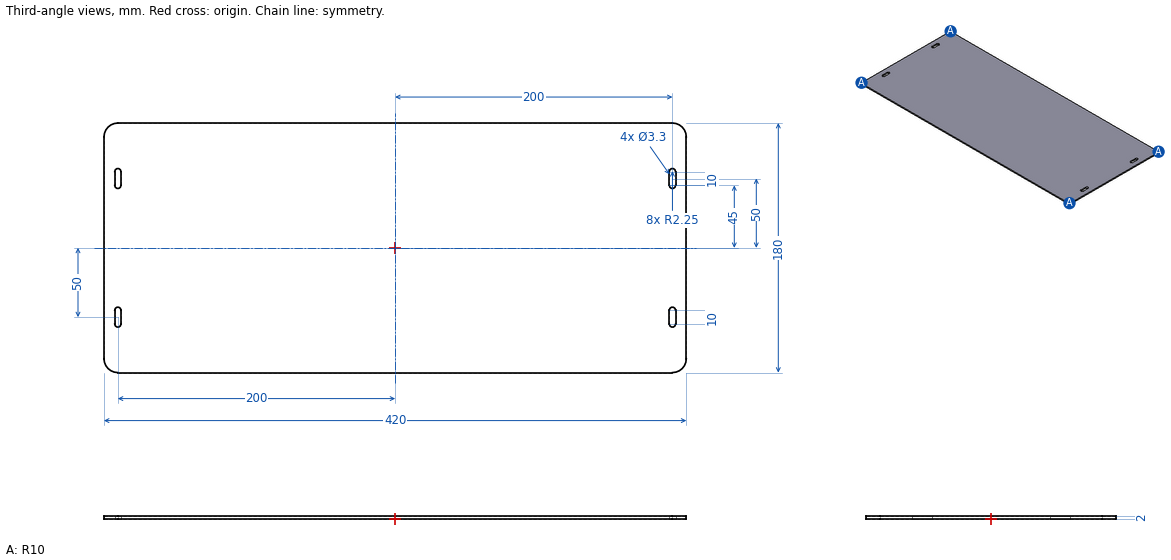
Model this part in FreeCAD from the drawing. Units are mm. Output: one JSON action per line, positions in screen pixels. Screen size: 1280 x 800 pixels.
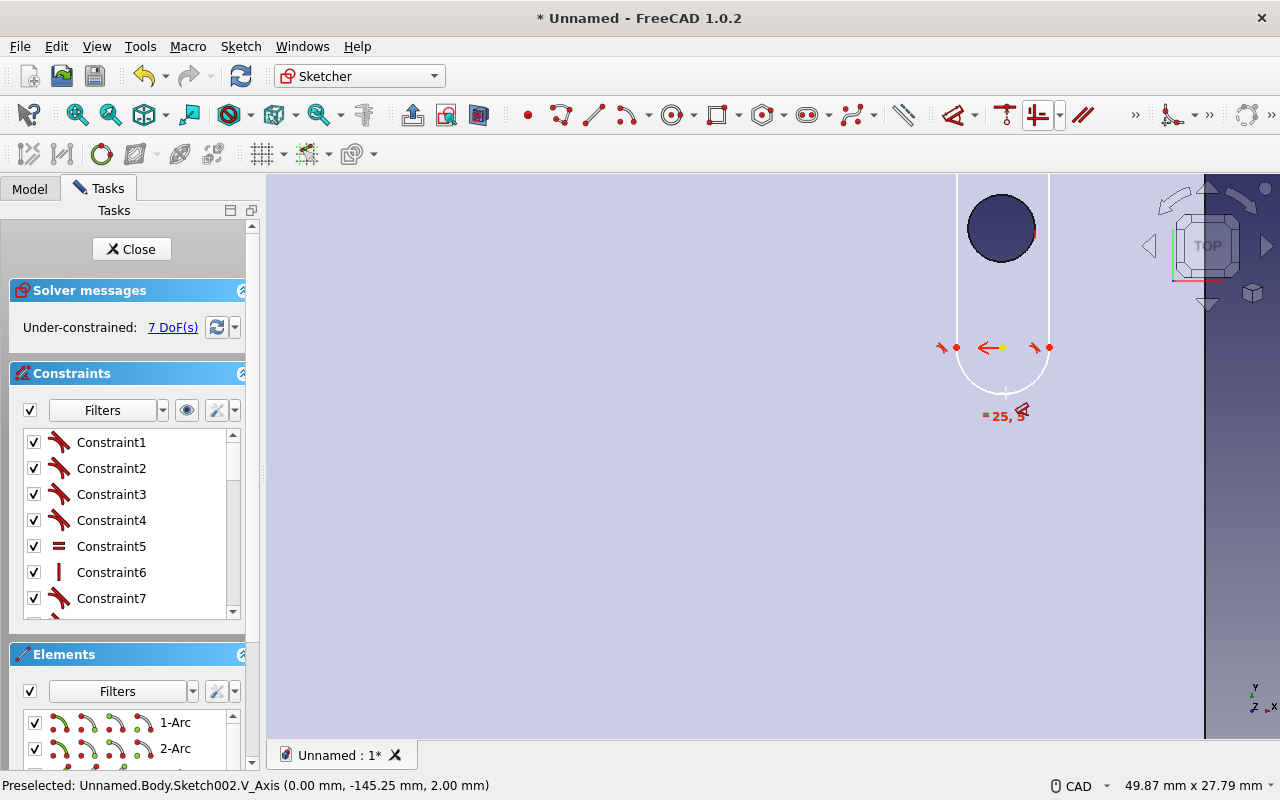
{"action": "left_click", "coordinate": [1003, 394]}
{"action": "left_click", "coordinate": [1003, 426]}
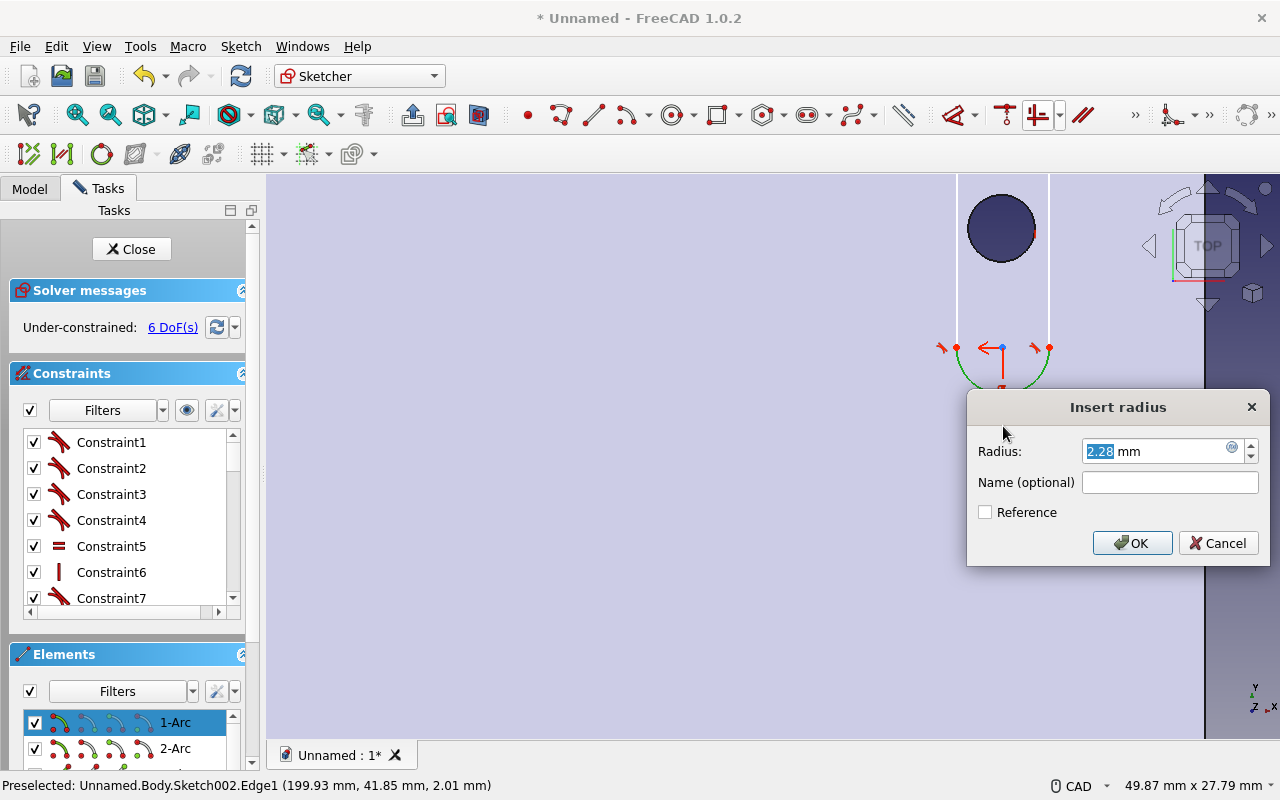
{"action": "type", "text": "2.25"}
{"action": "key", "text": "Return"}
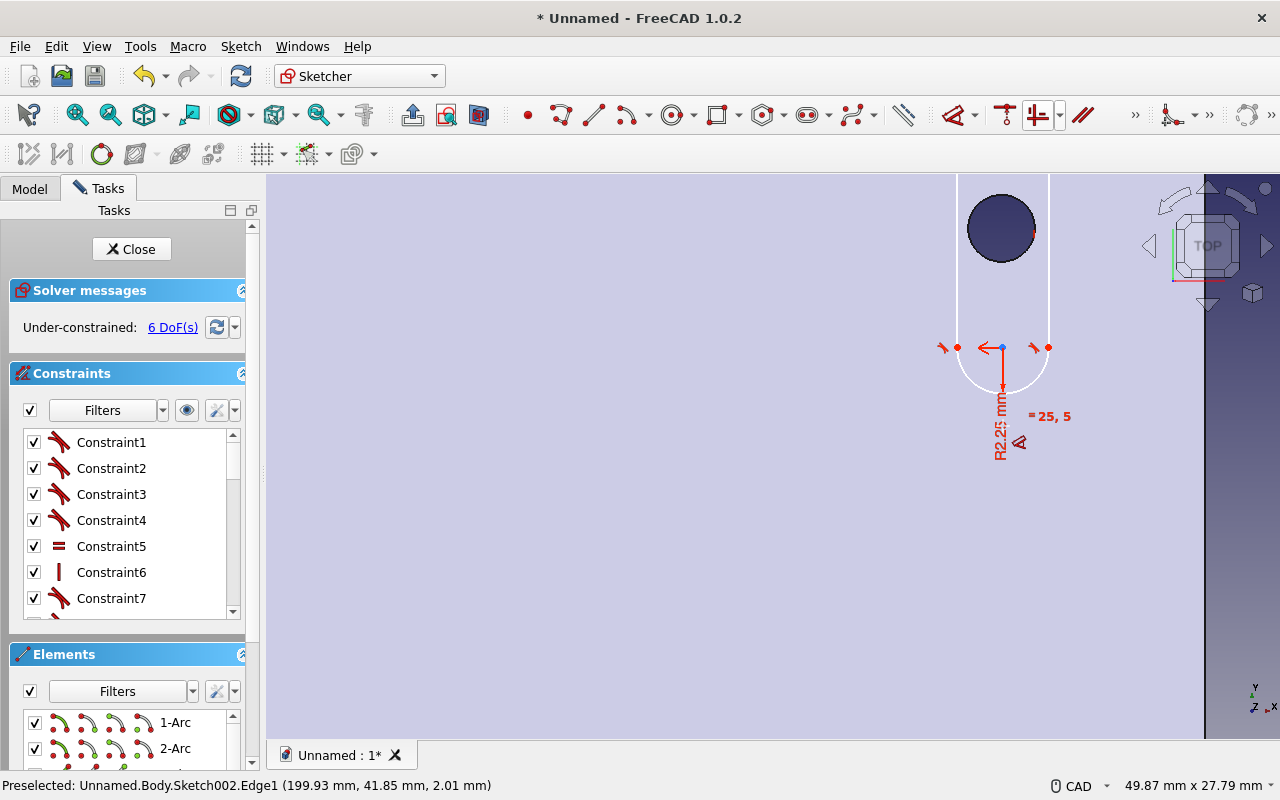
{"action": "scroll", "coordinate": [1007, 393], "scroll_direction": "down", "scroll_amount": 13}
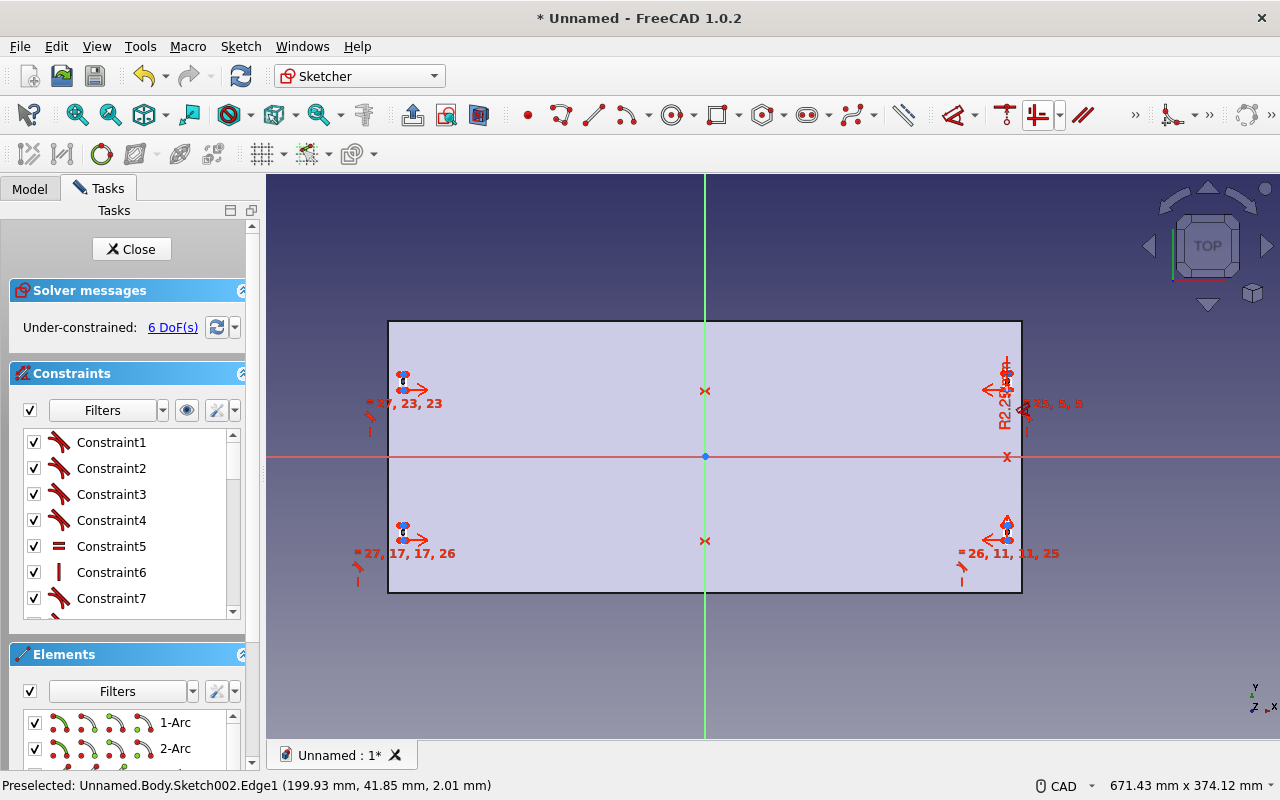
{"action": "scroll", "coordinate": [1004, 385], "scroll_direction": "up", "scroll_amount": 5}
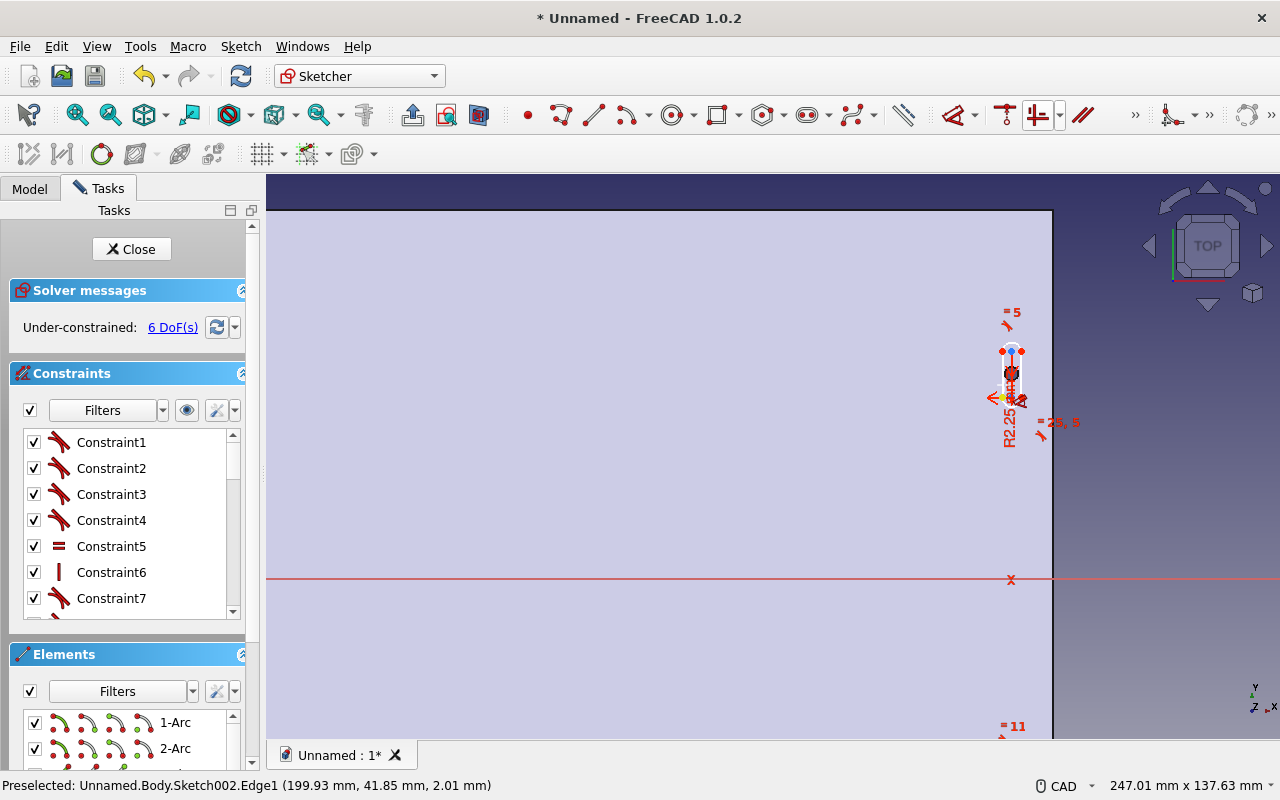
{"action": "left_click", "coordinate": [1003, 384]}
{"action": "left_click", "coordinate": [1037, 375]}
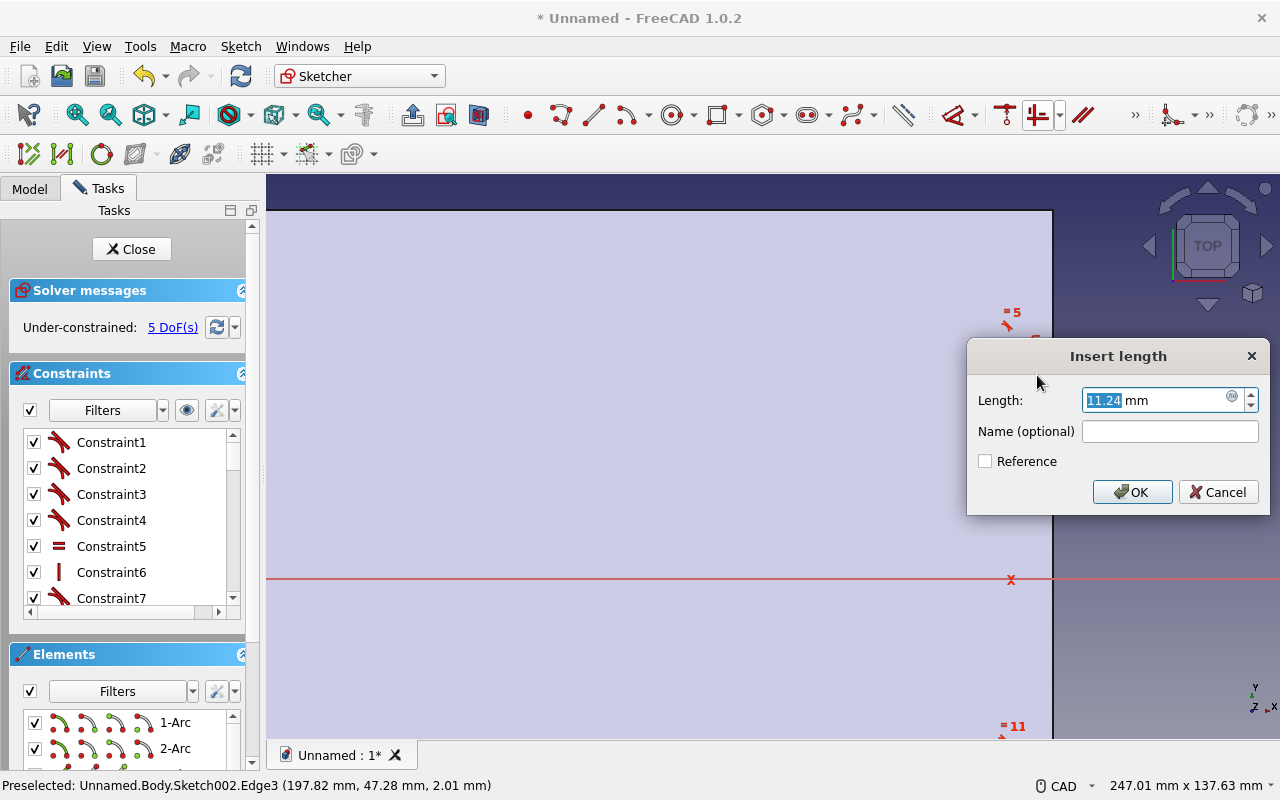
{"action": "type", "text": "10"}
{"action": "key", "text": "Return"}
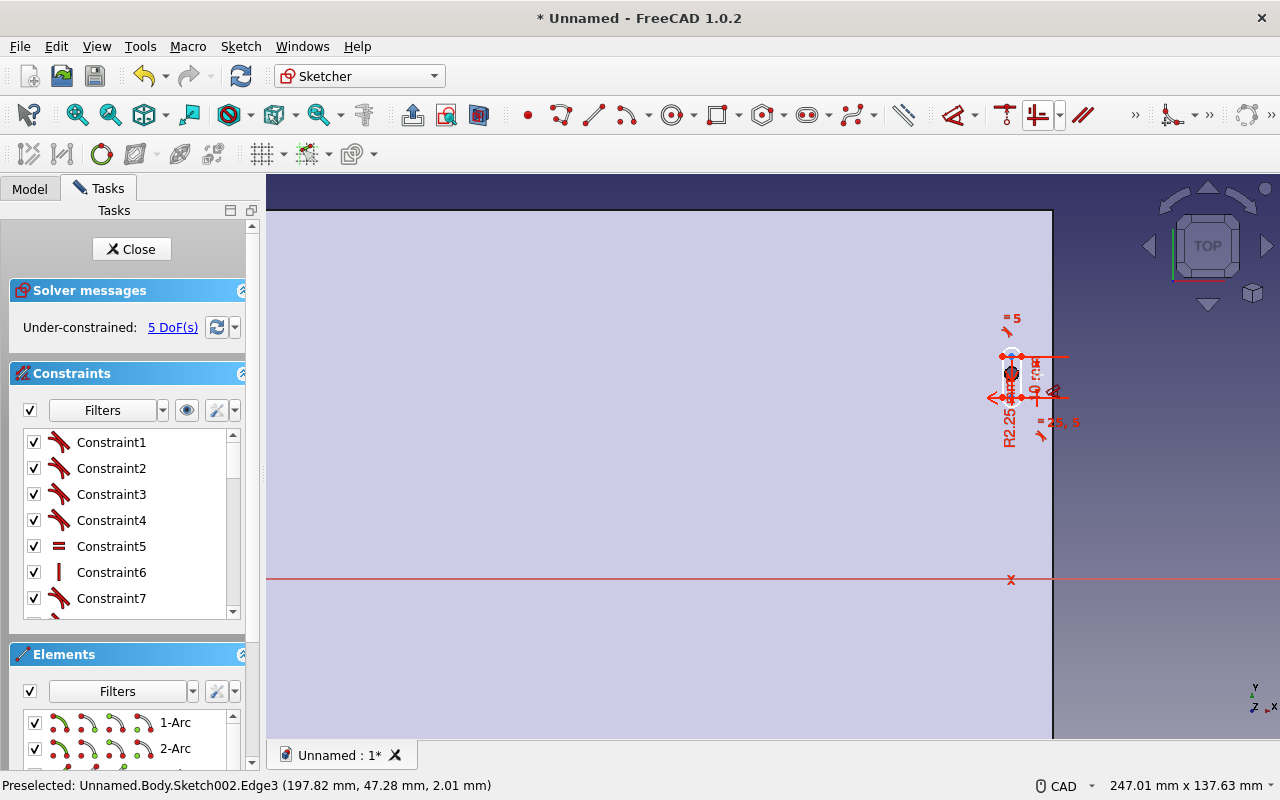
{"action": "scroll", "coordinate": [1004, 385], "scroll_direction": "down", "scroll_amount": 5}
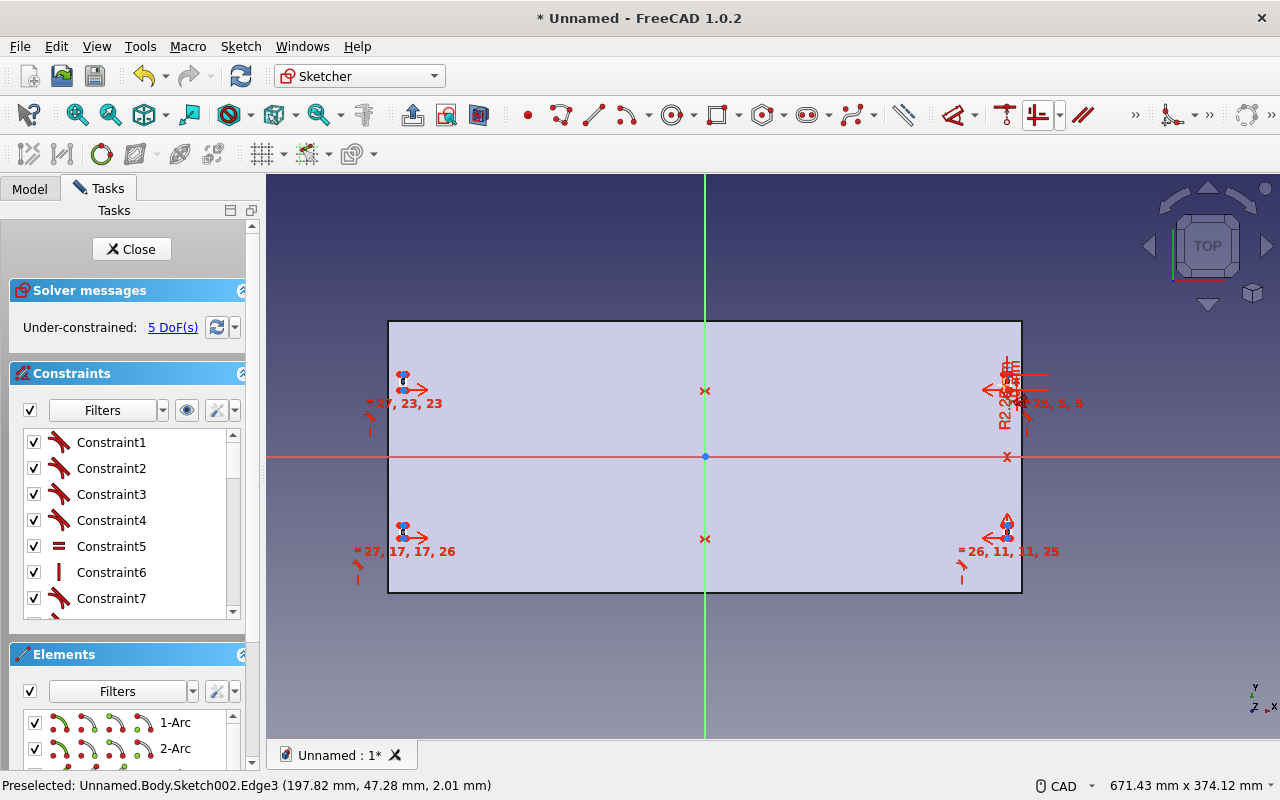
{"action": "scroll", "coordinate": [1004, 534], "scroll_direction": "up", "scroll_amount": 7}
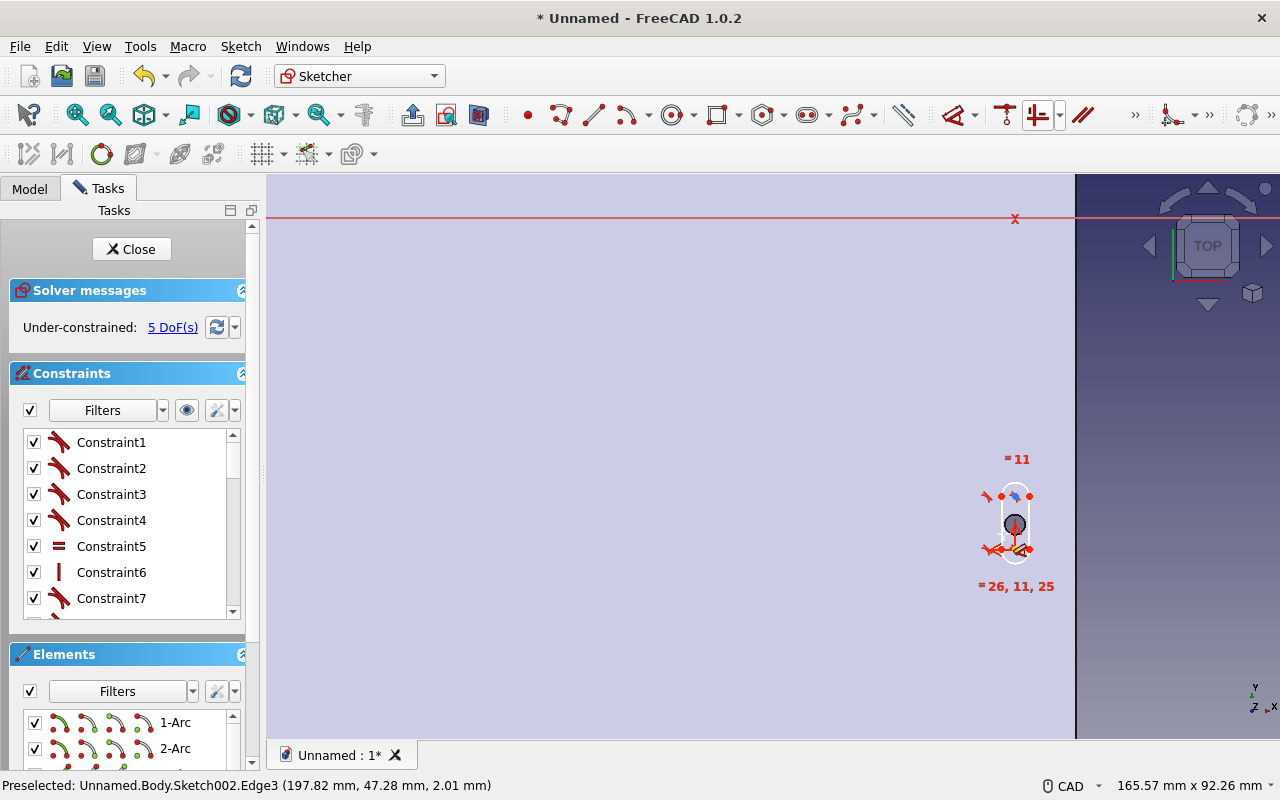
{"action": "left_click", "coordinate": [1002, 534]}
{"action": "left_click", "coordinate": [968, 523]}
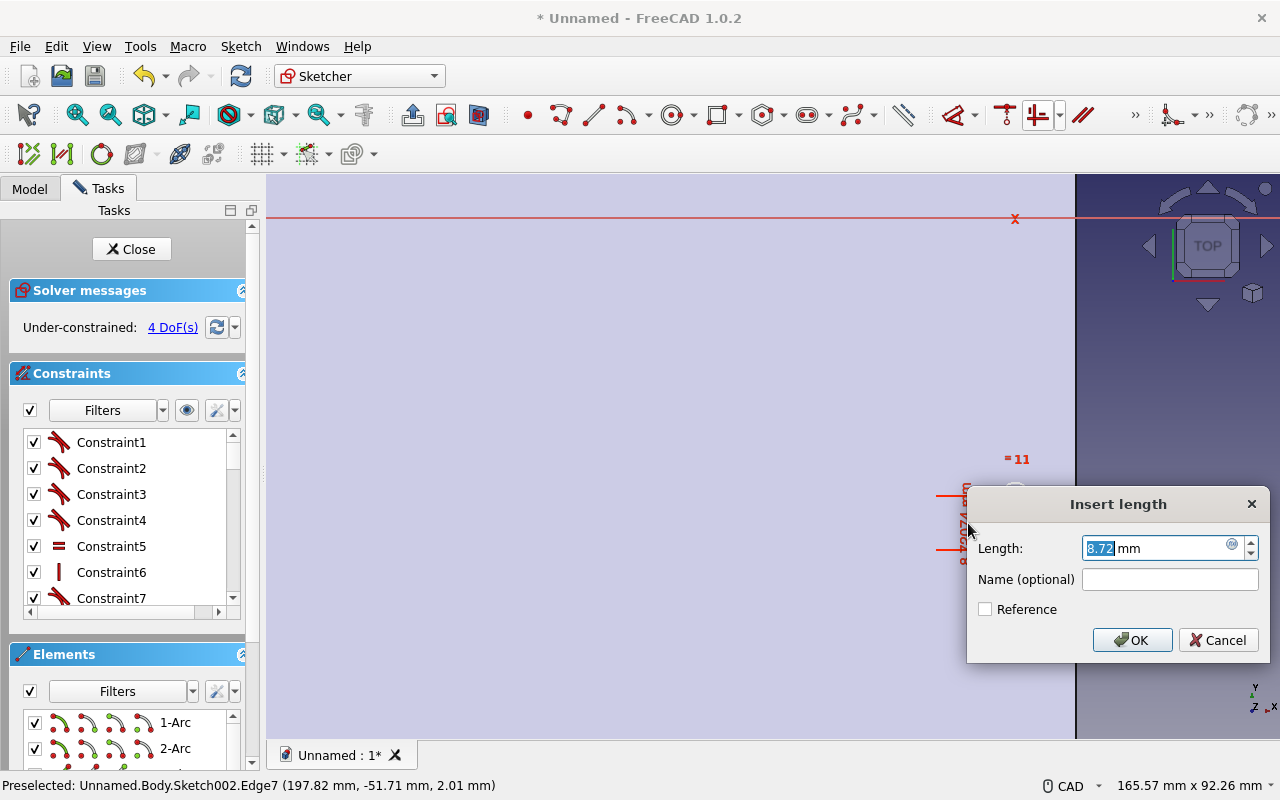
{"action": "type", "text": "10"}
{"action": "key", "text": "Return"}